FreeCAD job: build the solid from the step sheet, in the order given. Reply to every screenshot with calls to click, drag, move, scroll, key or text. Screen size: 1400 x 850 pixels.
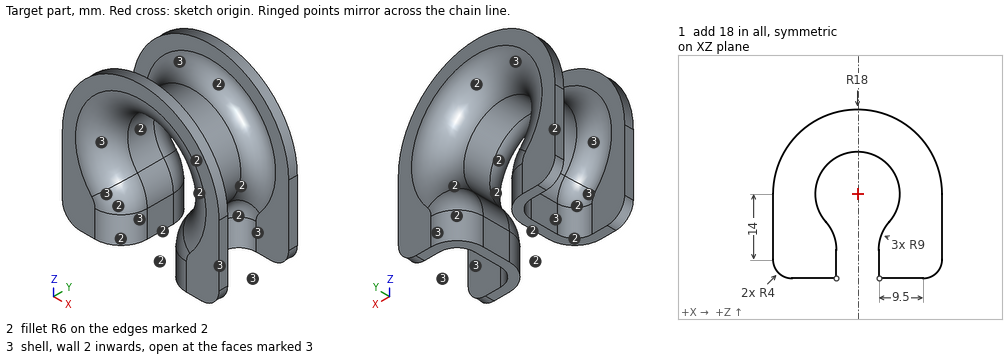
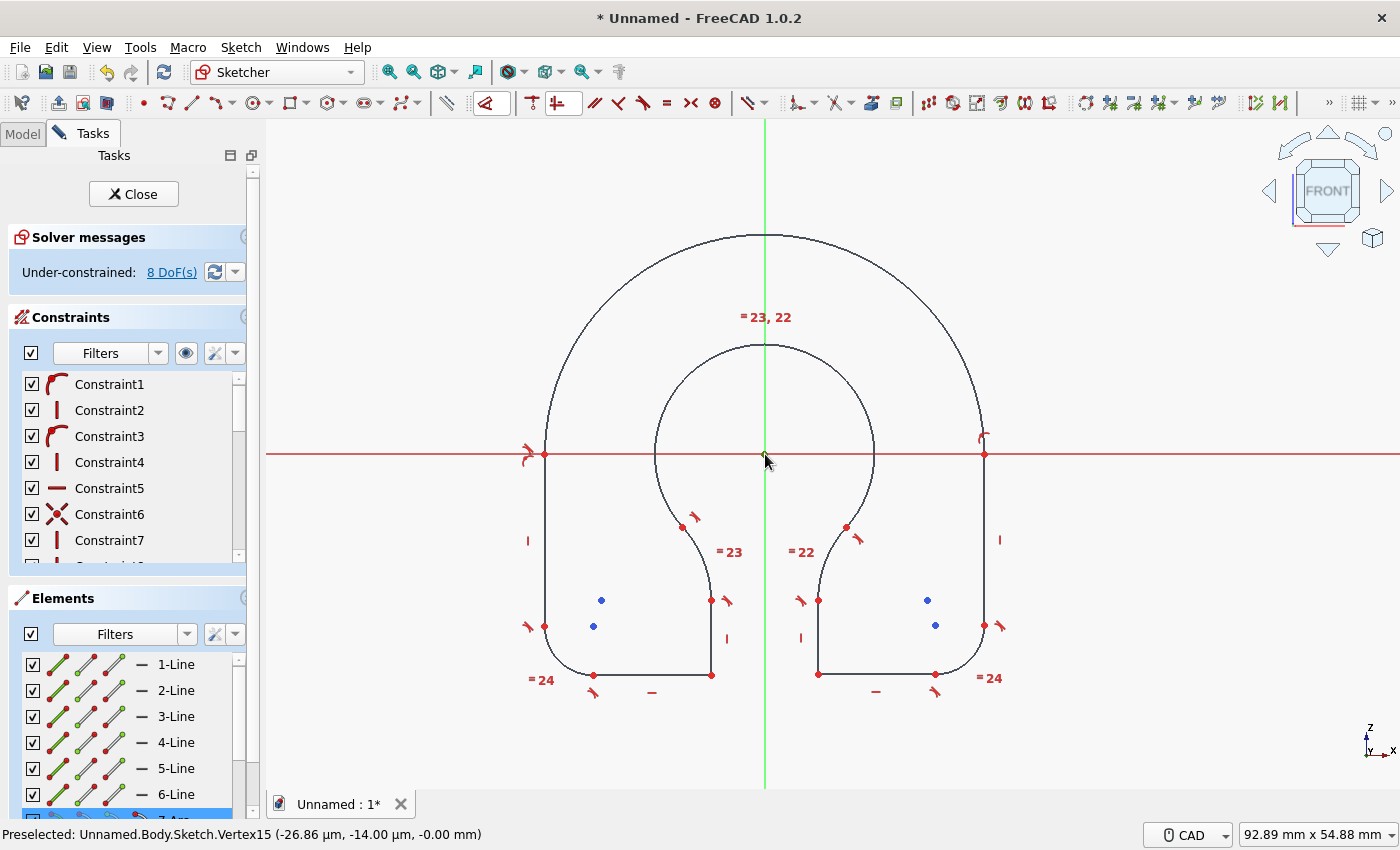
click(765, 717)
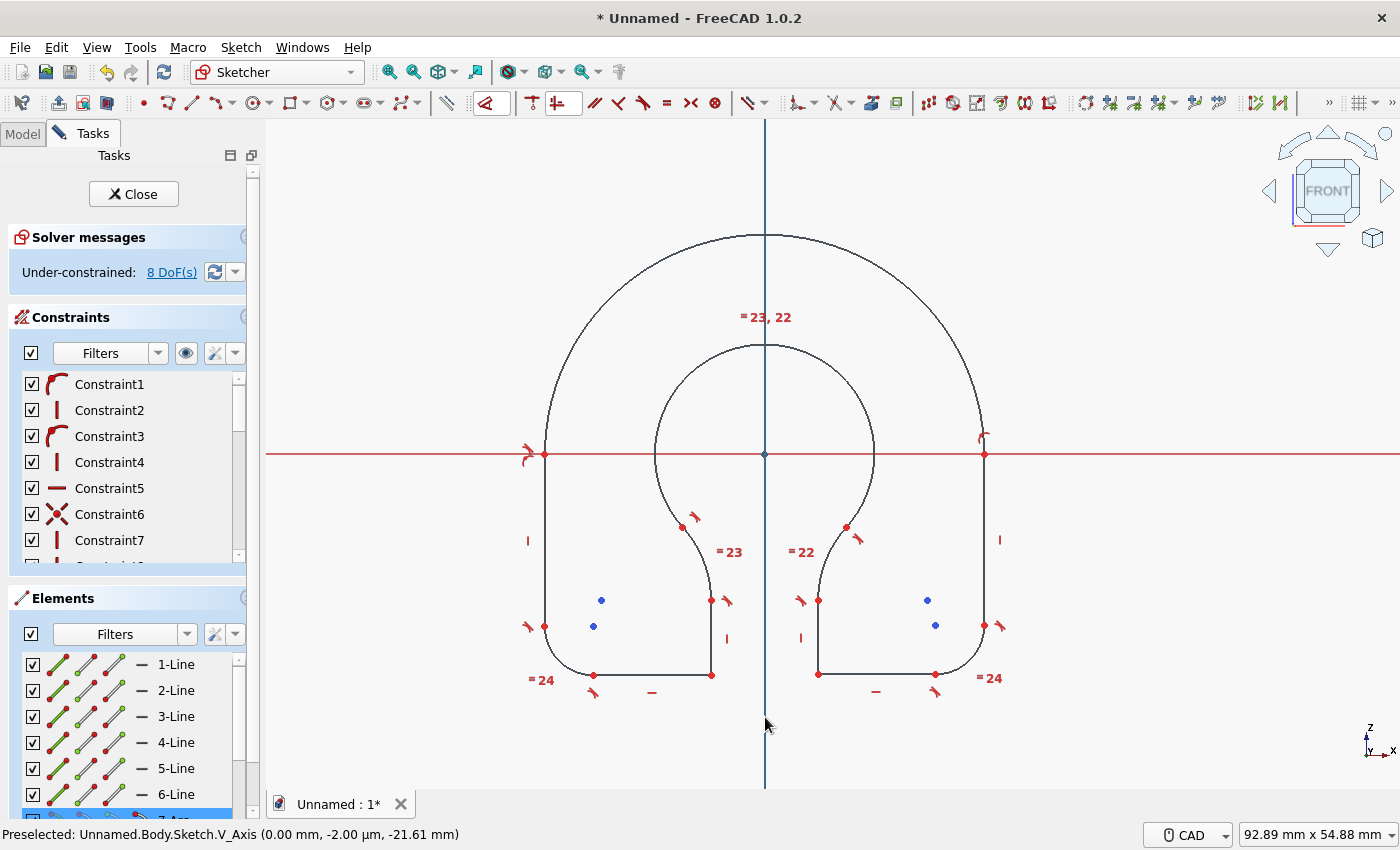
key(c)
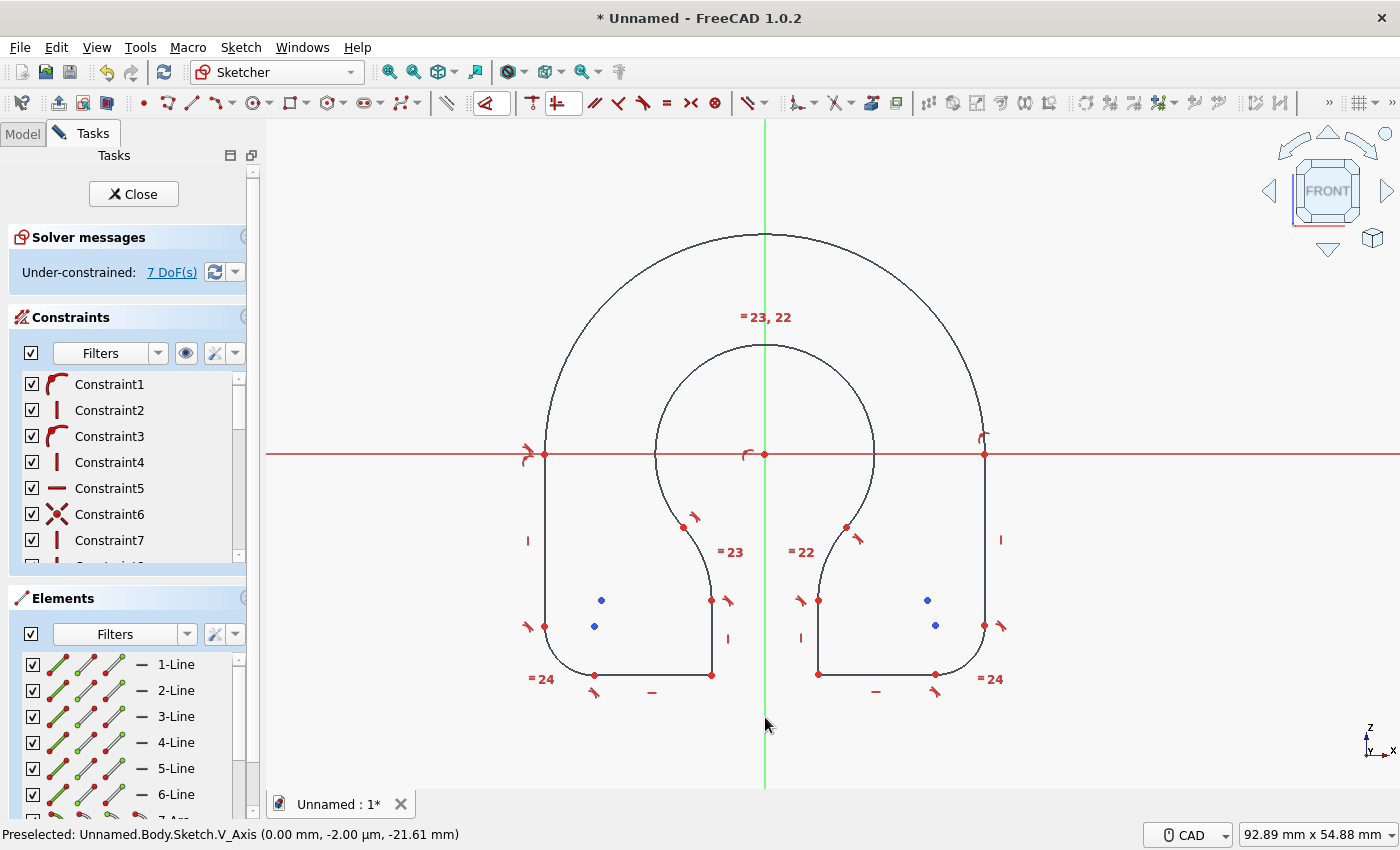
click(818, 675)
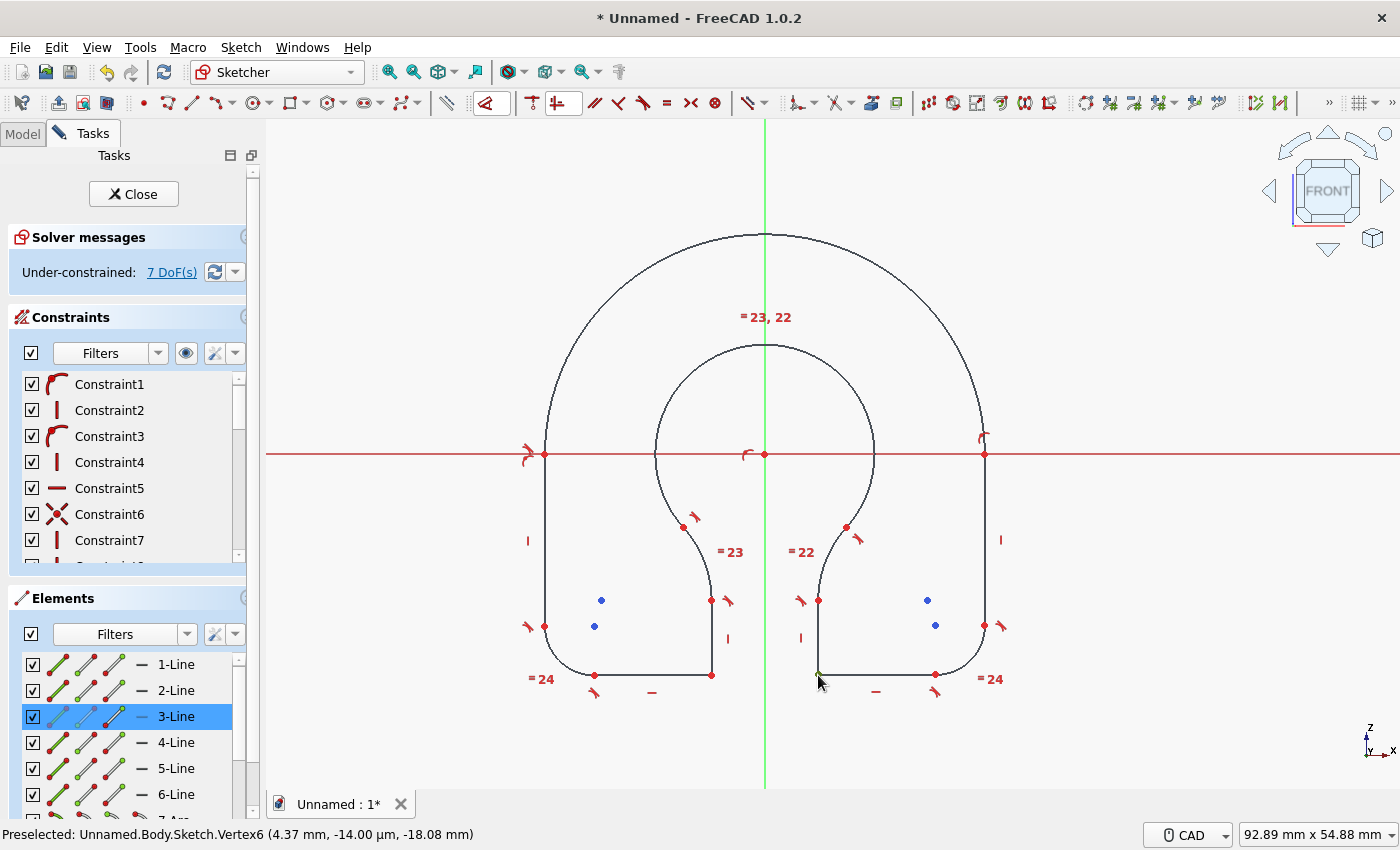
click(712, 675)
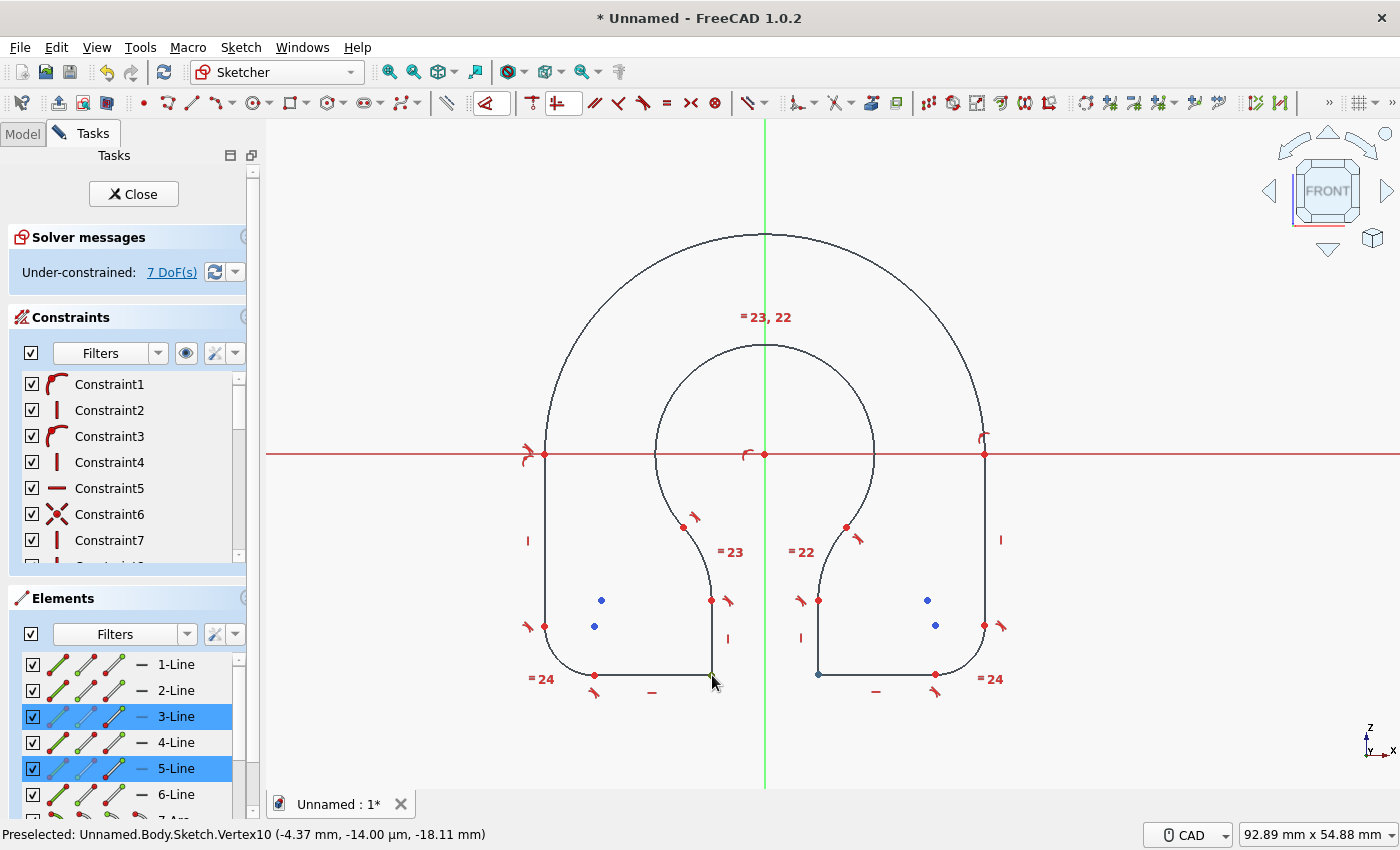
click(765, 717)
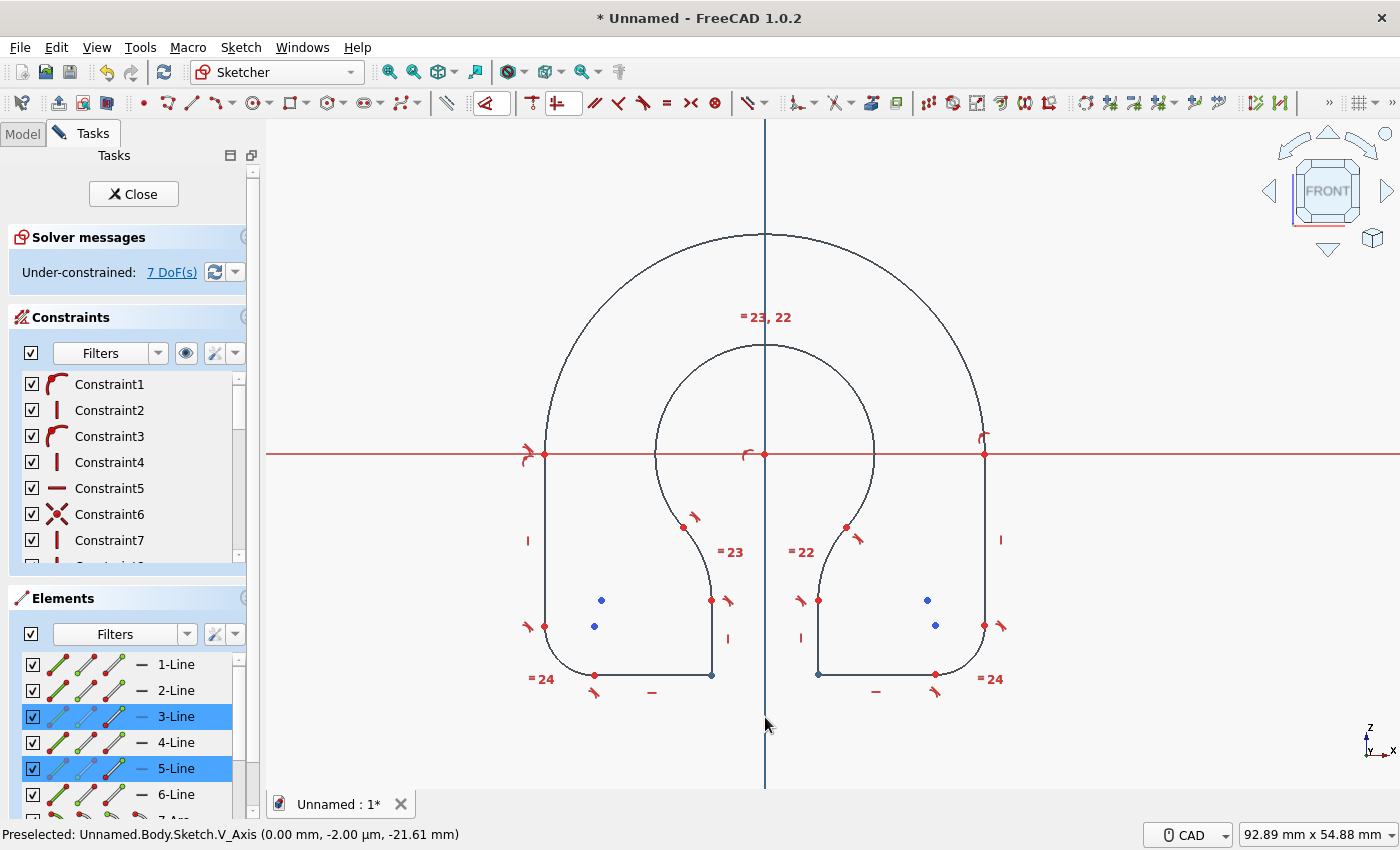
key(s)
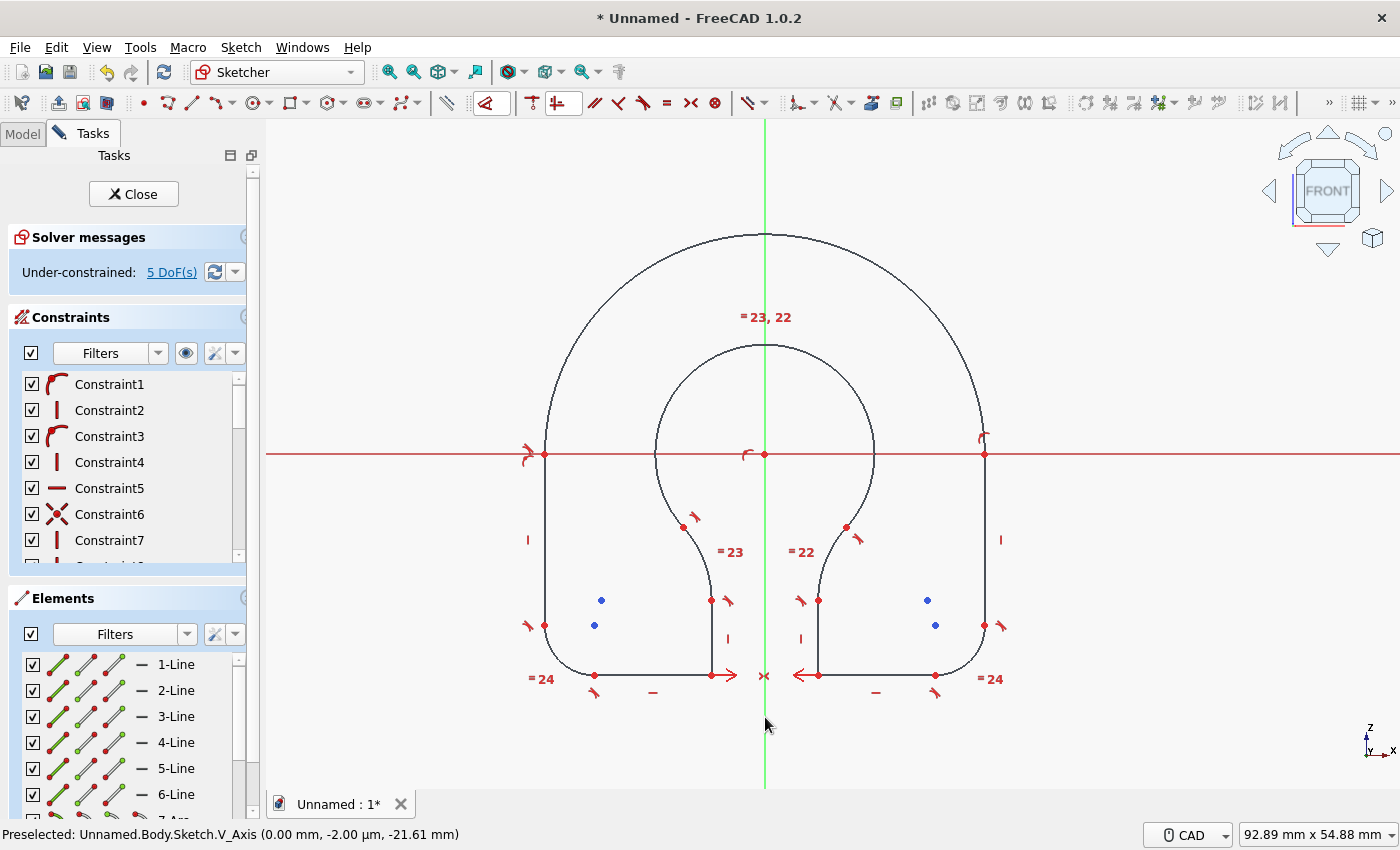
click(894, 276)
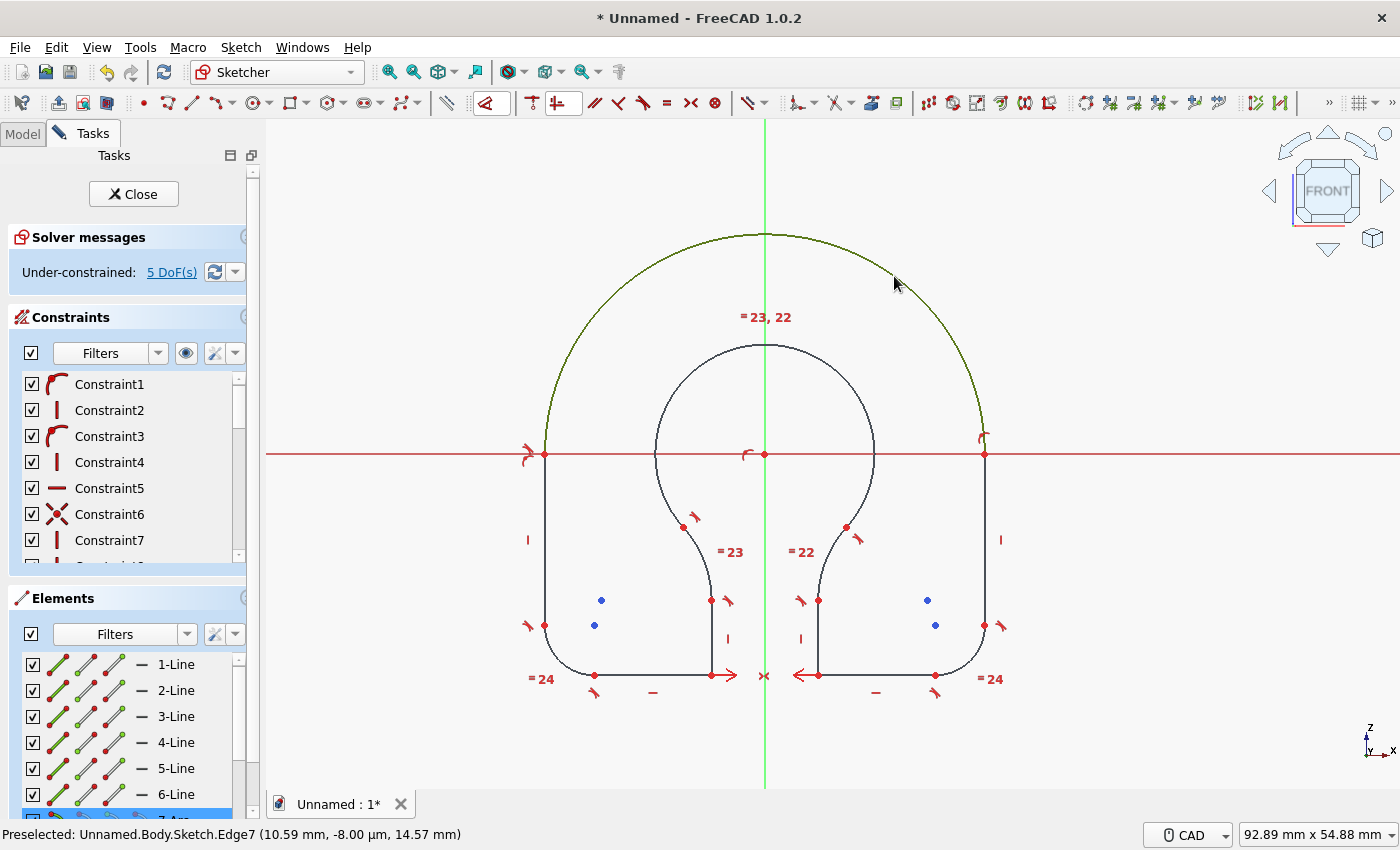
key(k)
key(r)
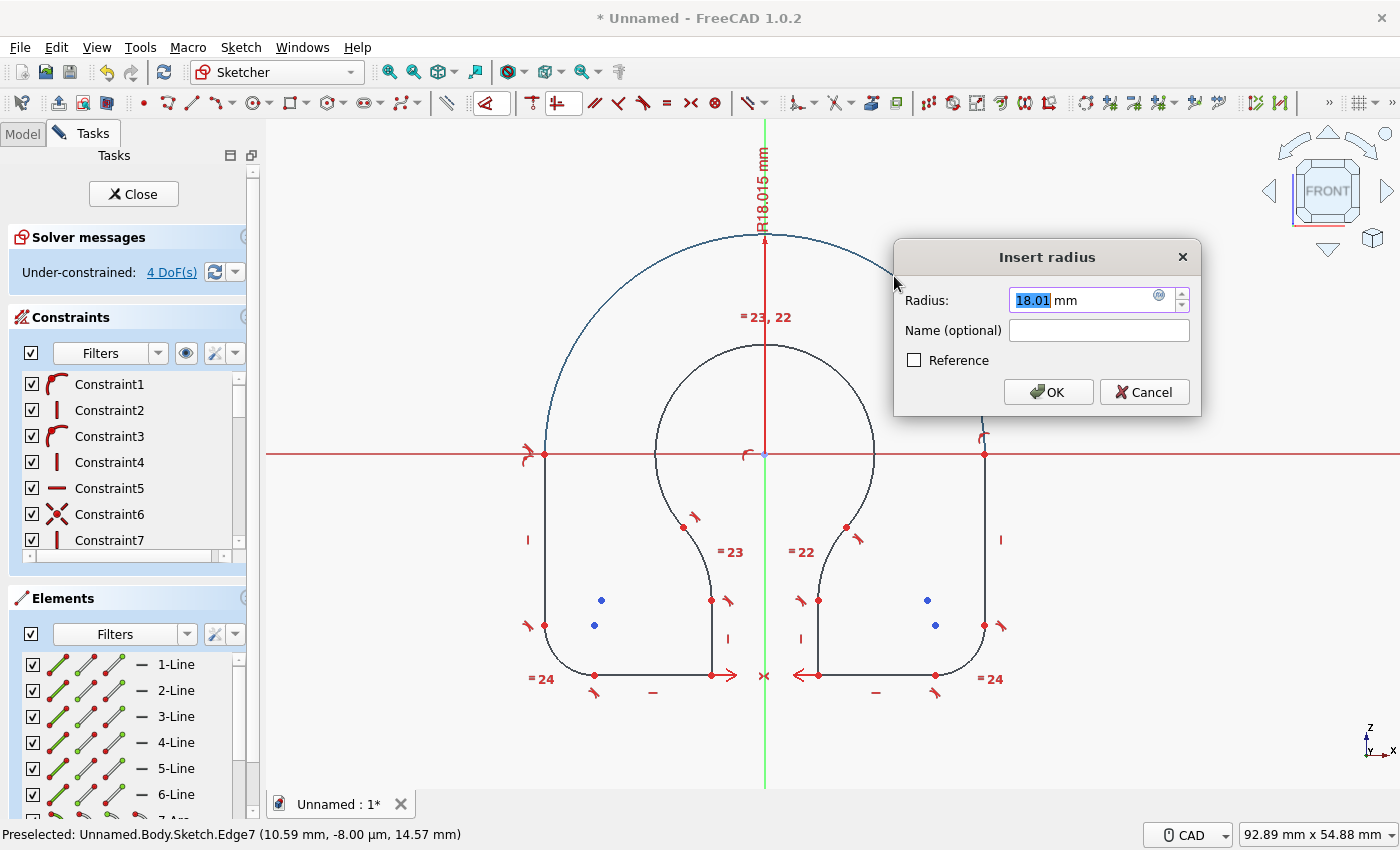
text(18)
key(Return)